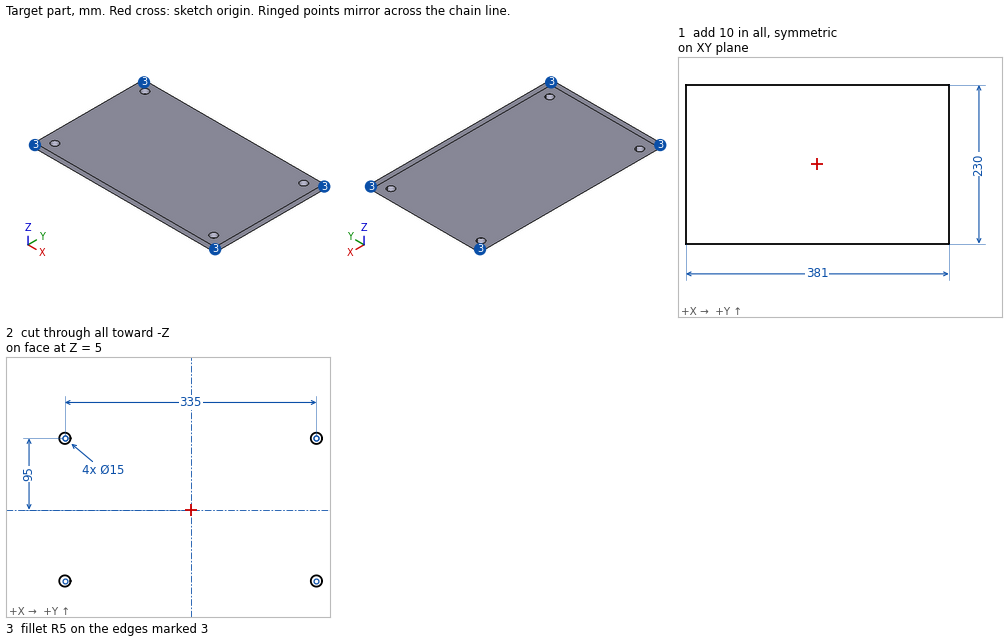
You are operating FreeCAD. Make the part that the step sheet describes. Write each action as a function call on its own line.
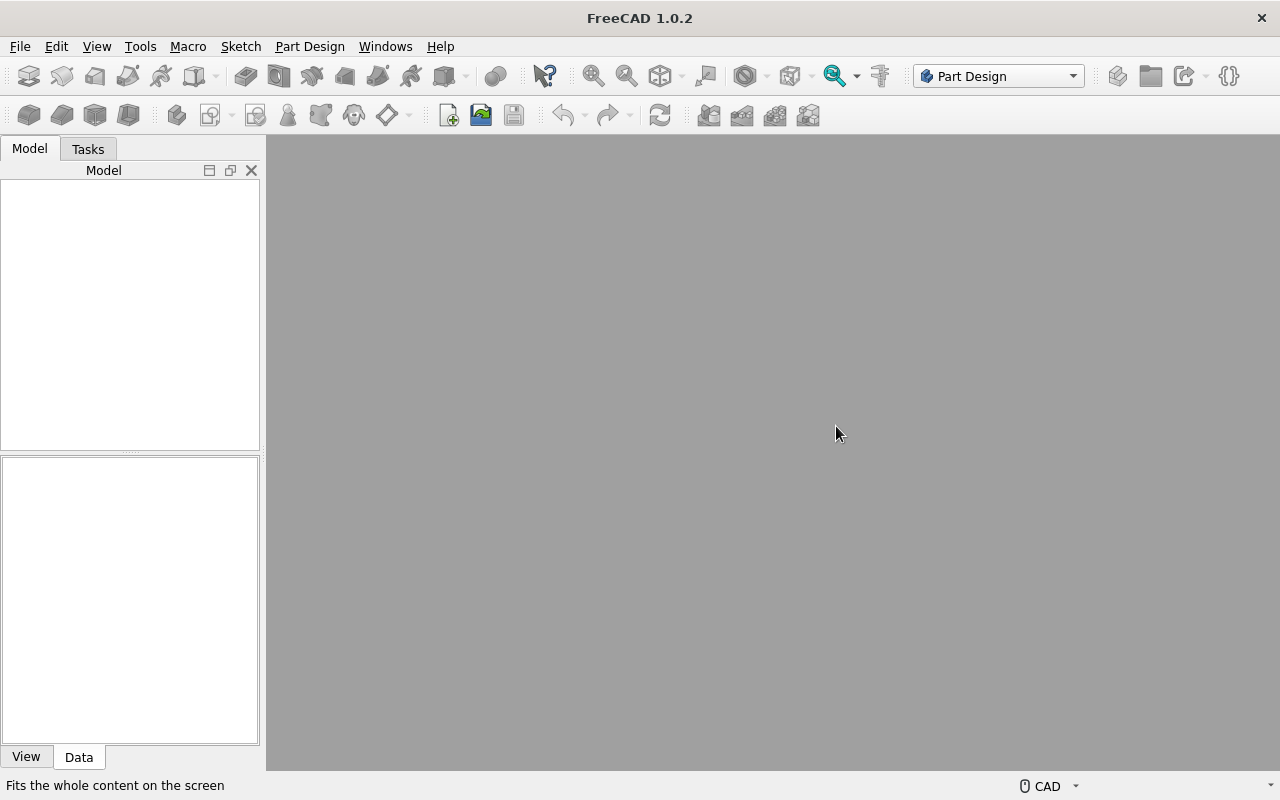
click(448, 116)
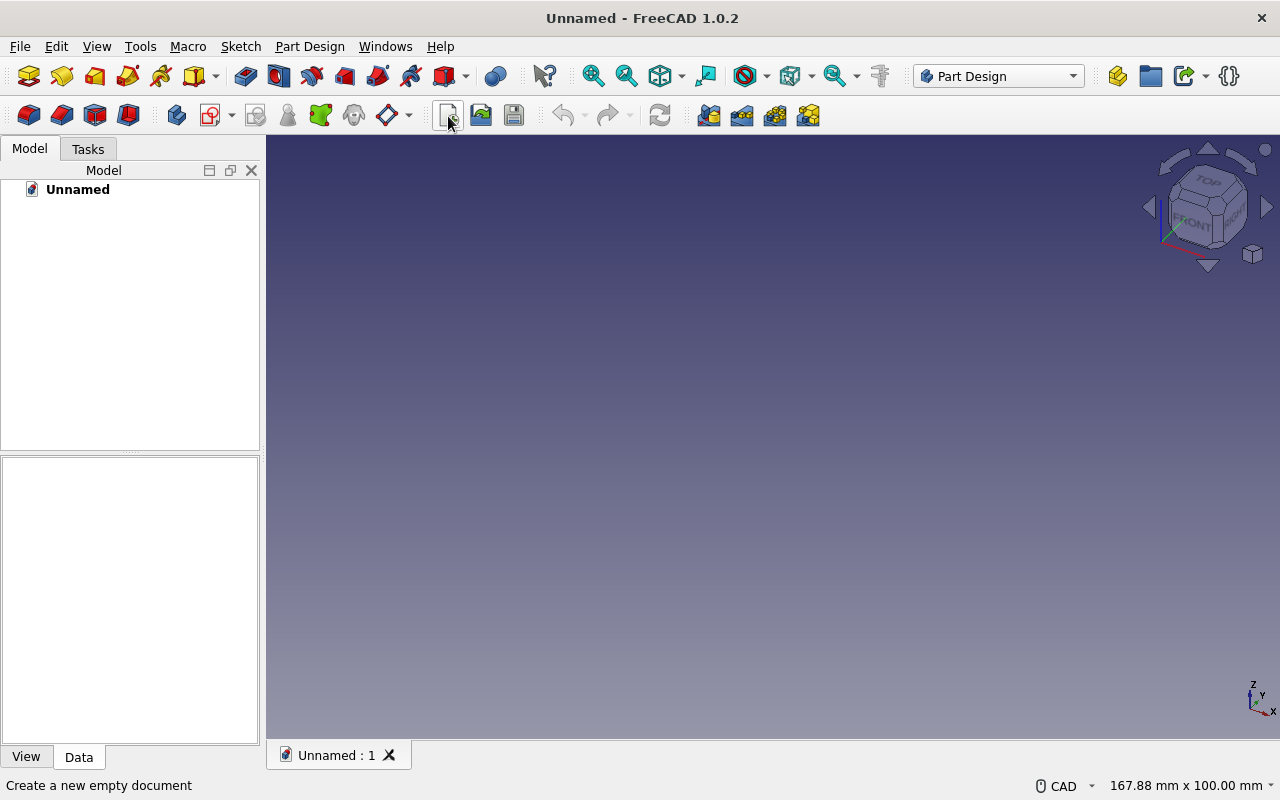
click(210, 116)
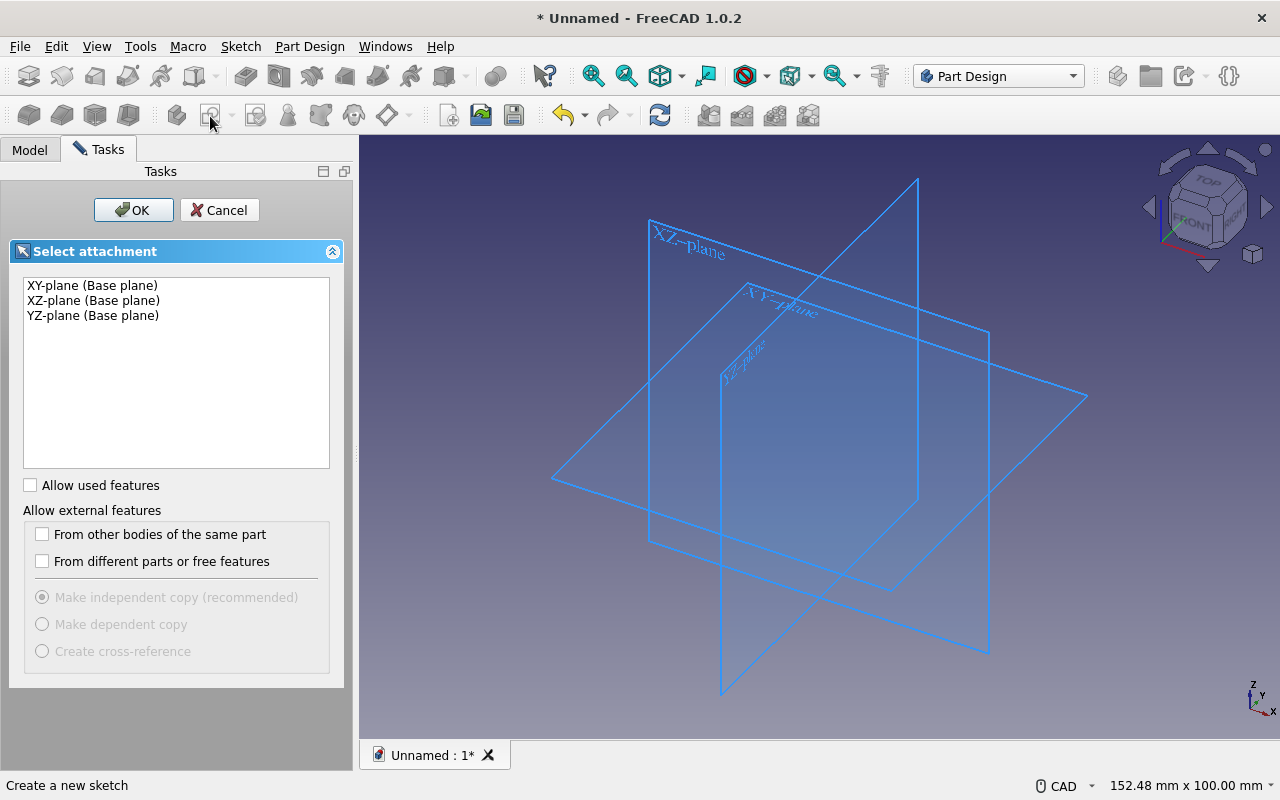
click(84, 286)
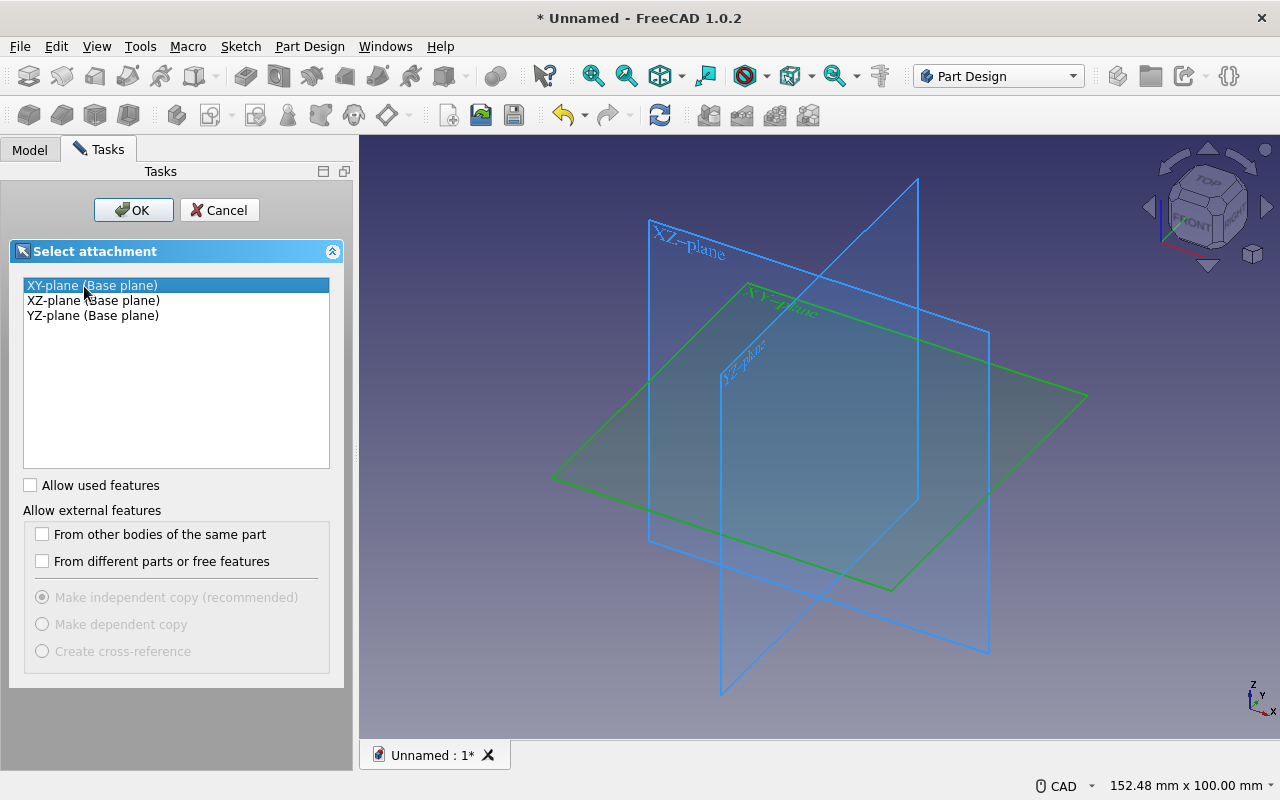
click(134, 210)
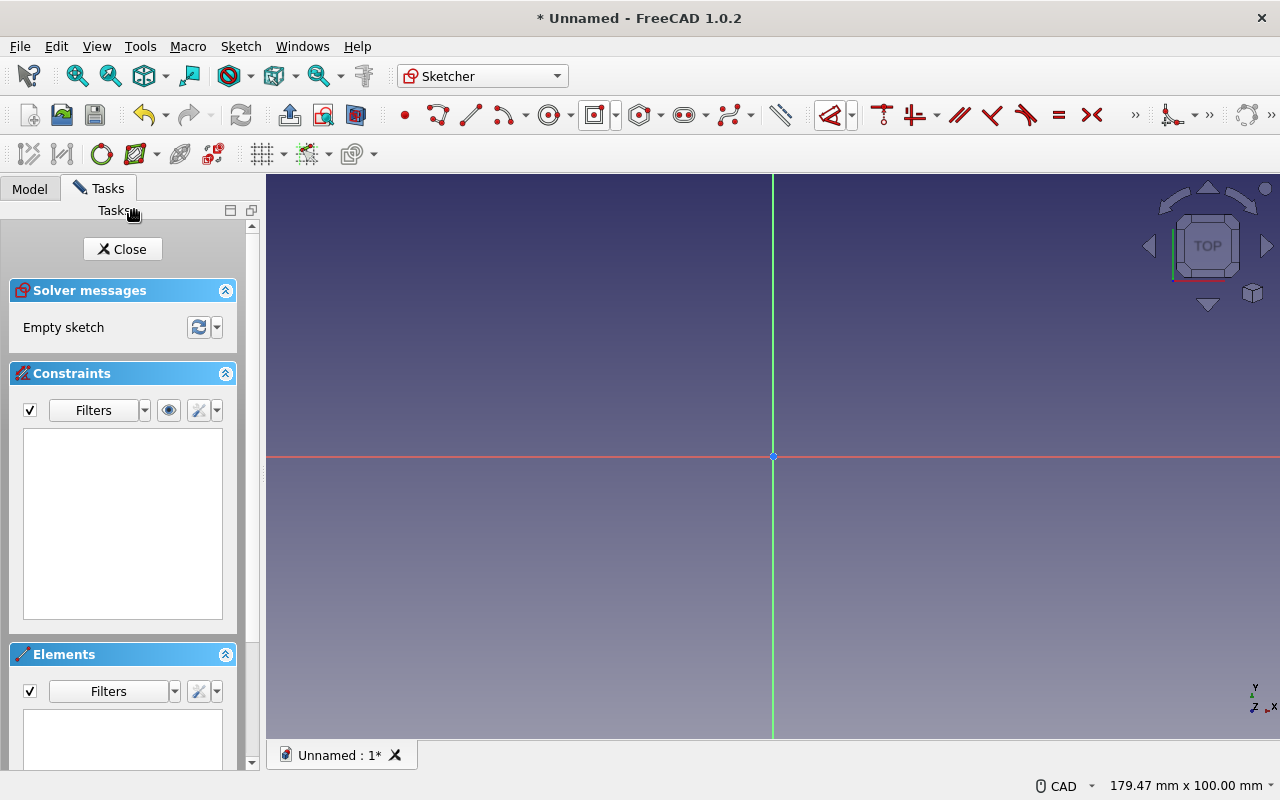
scroll(682, 456, down, 7)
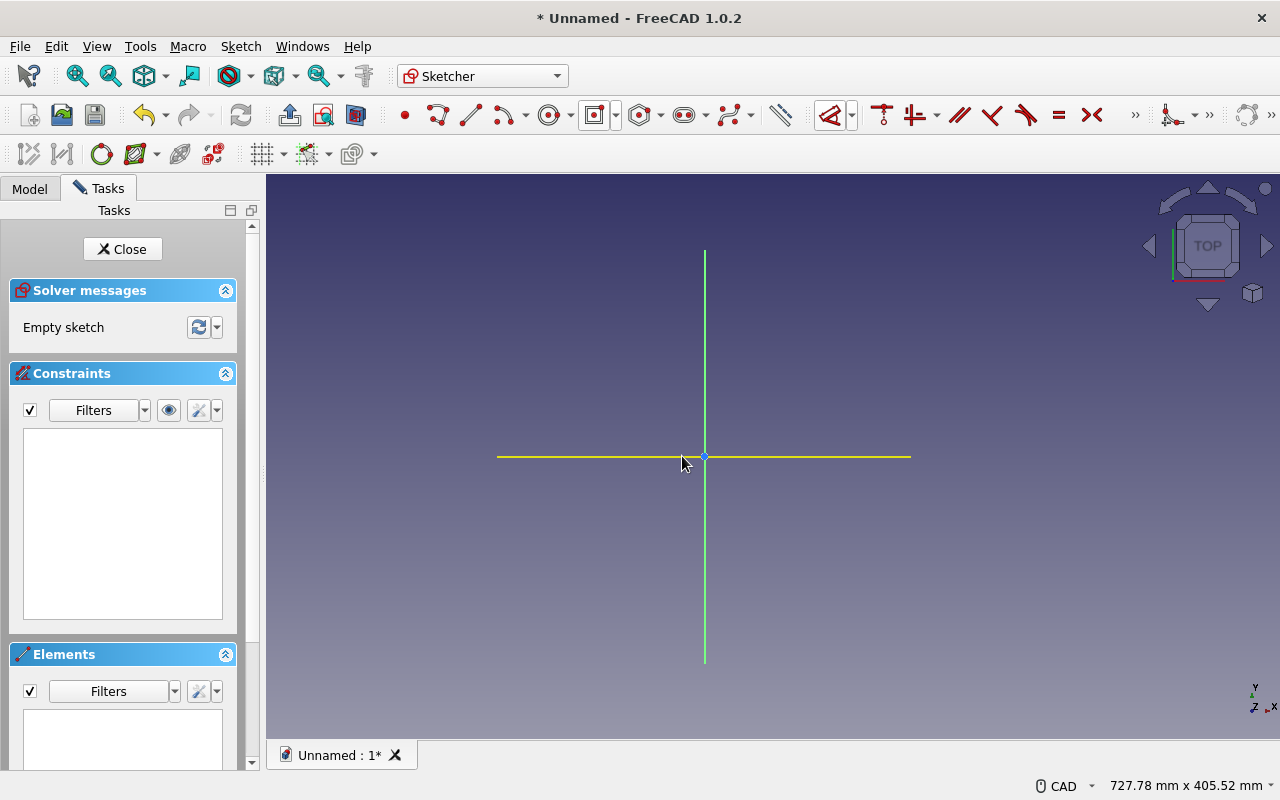
click(594, 116)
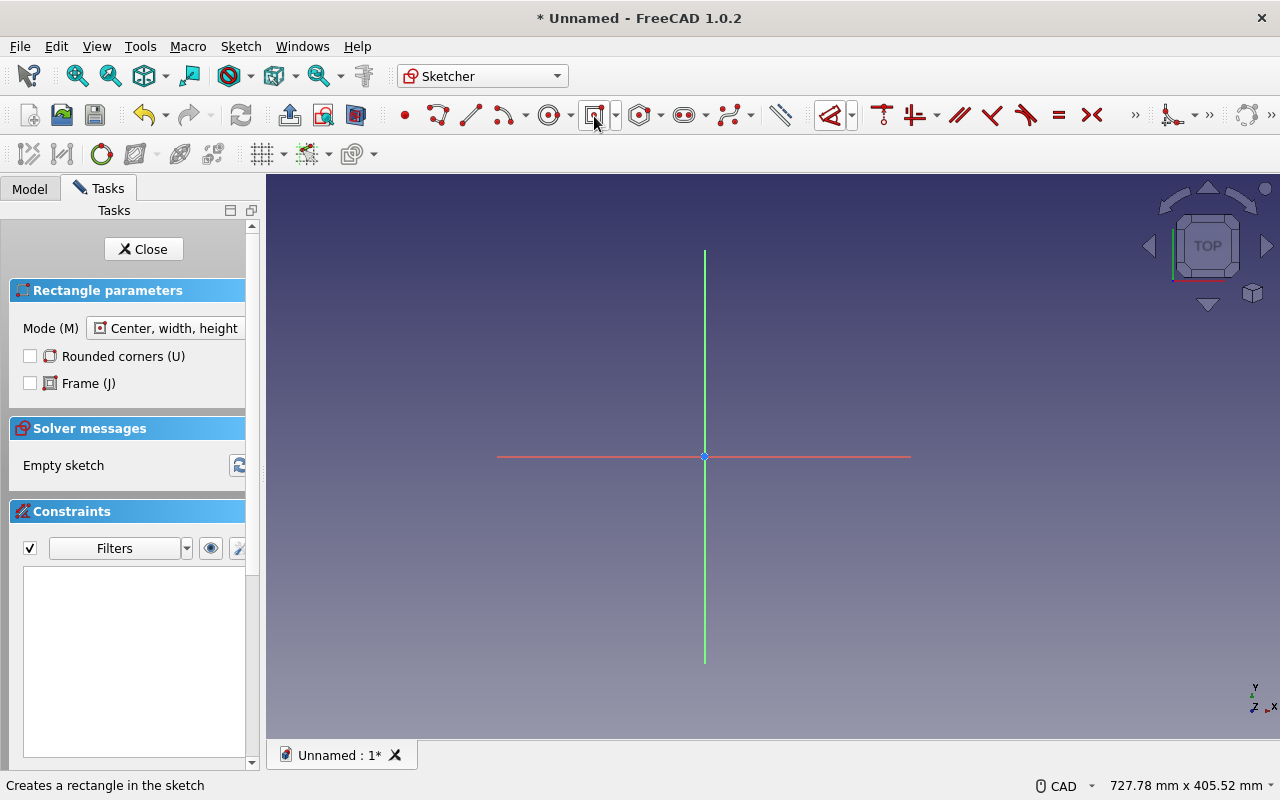
click(705, 456)
click(970, 296)
key(Escape)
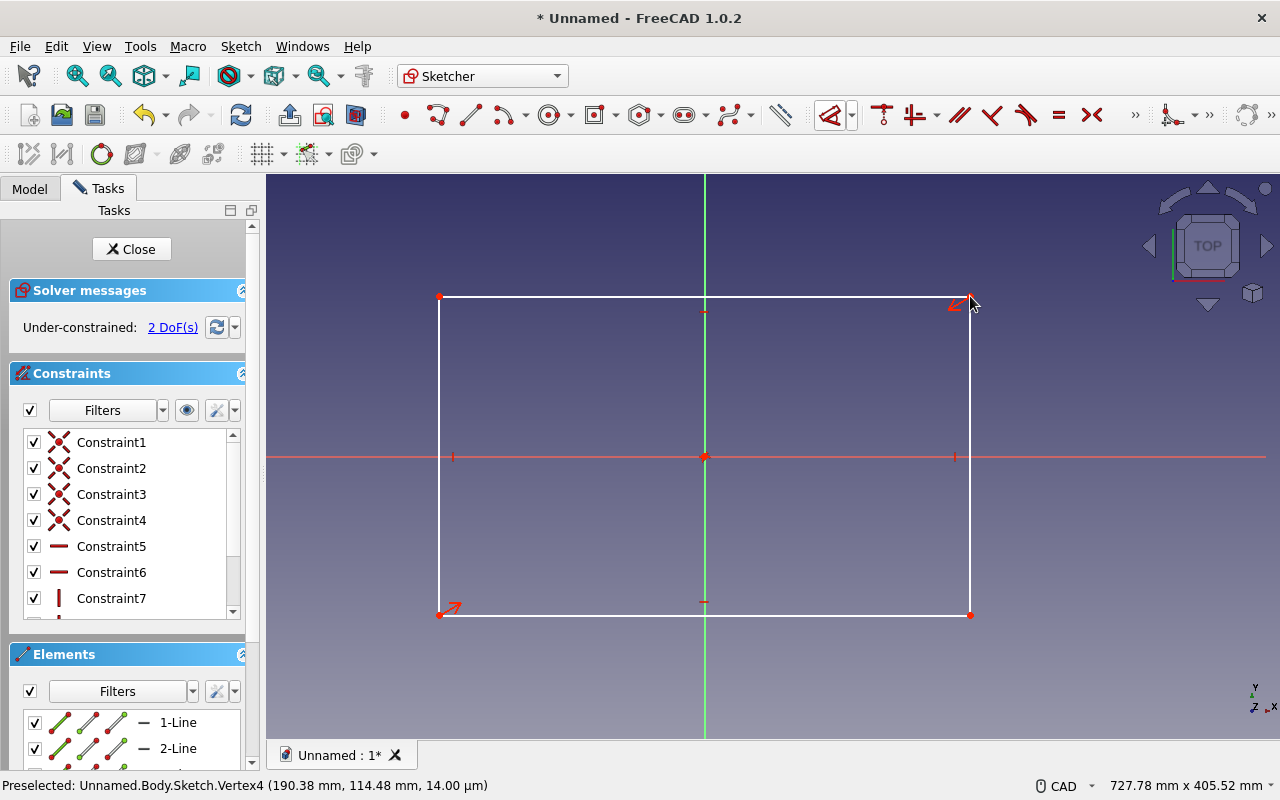
click(599, 616)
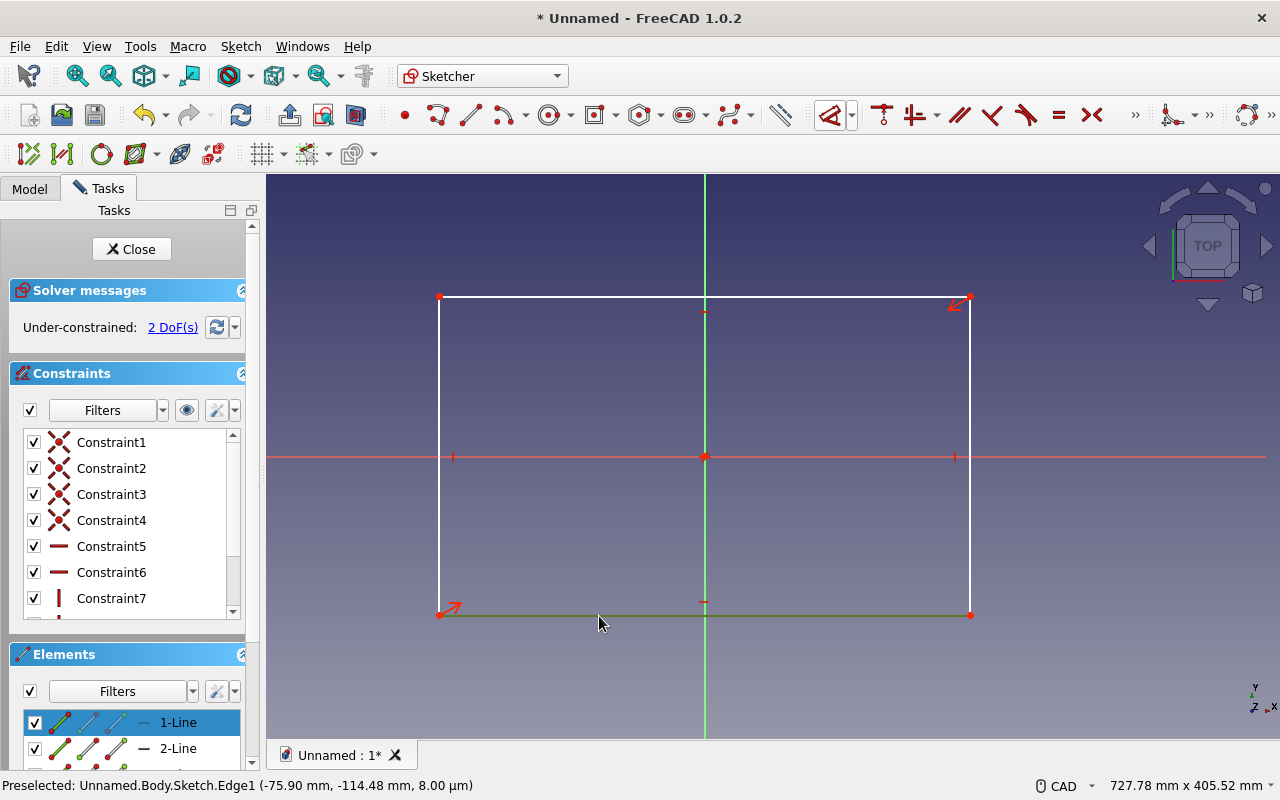
key(l)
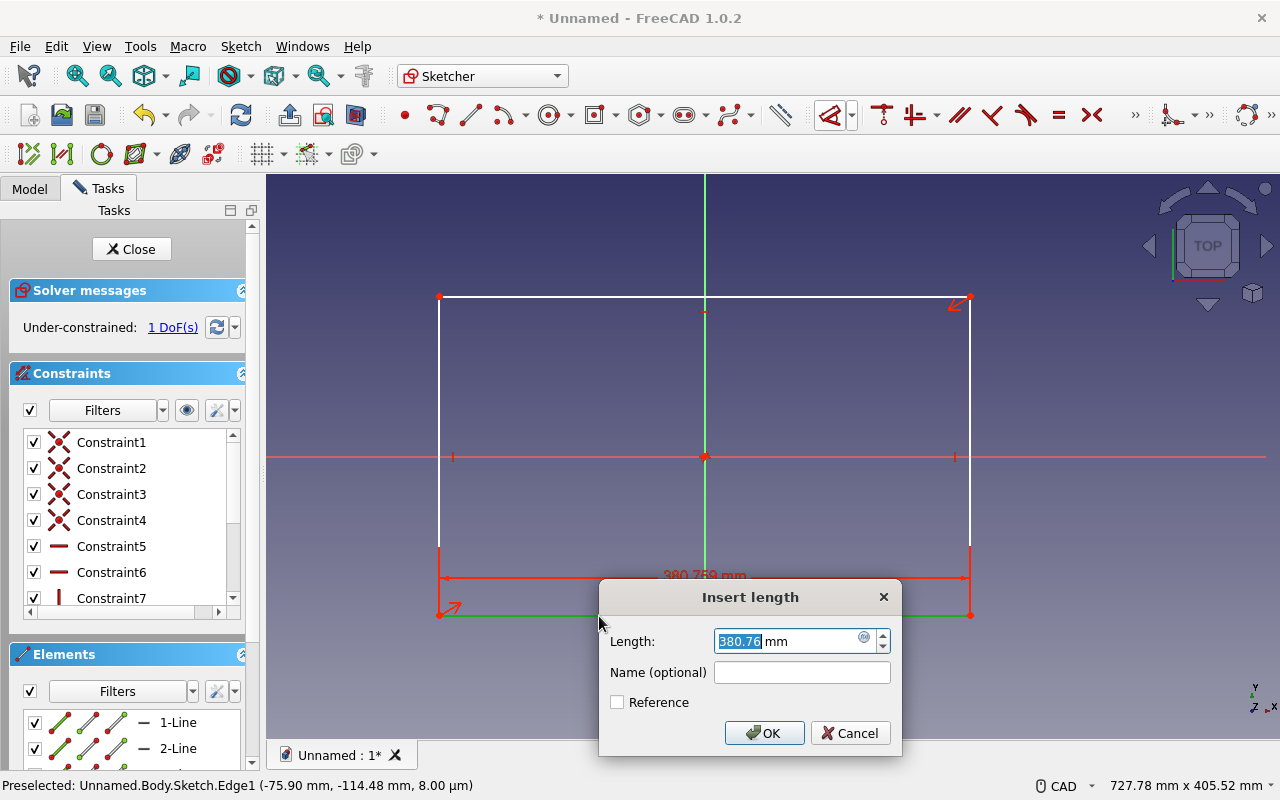
text(381)
key(Return)